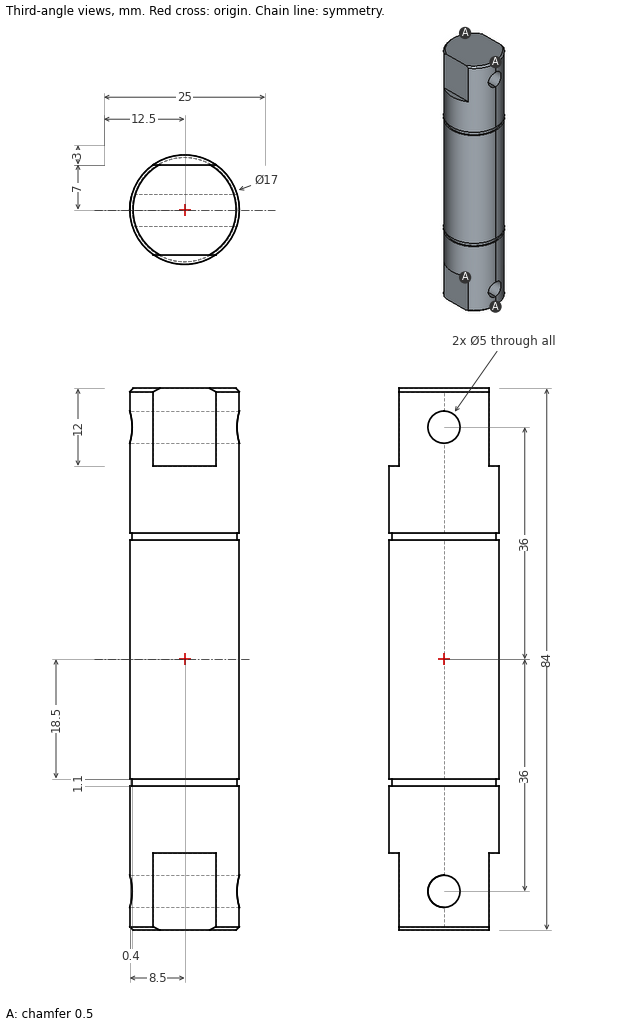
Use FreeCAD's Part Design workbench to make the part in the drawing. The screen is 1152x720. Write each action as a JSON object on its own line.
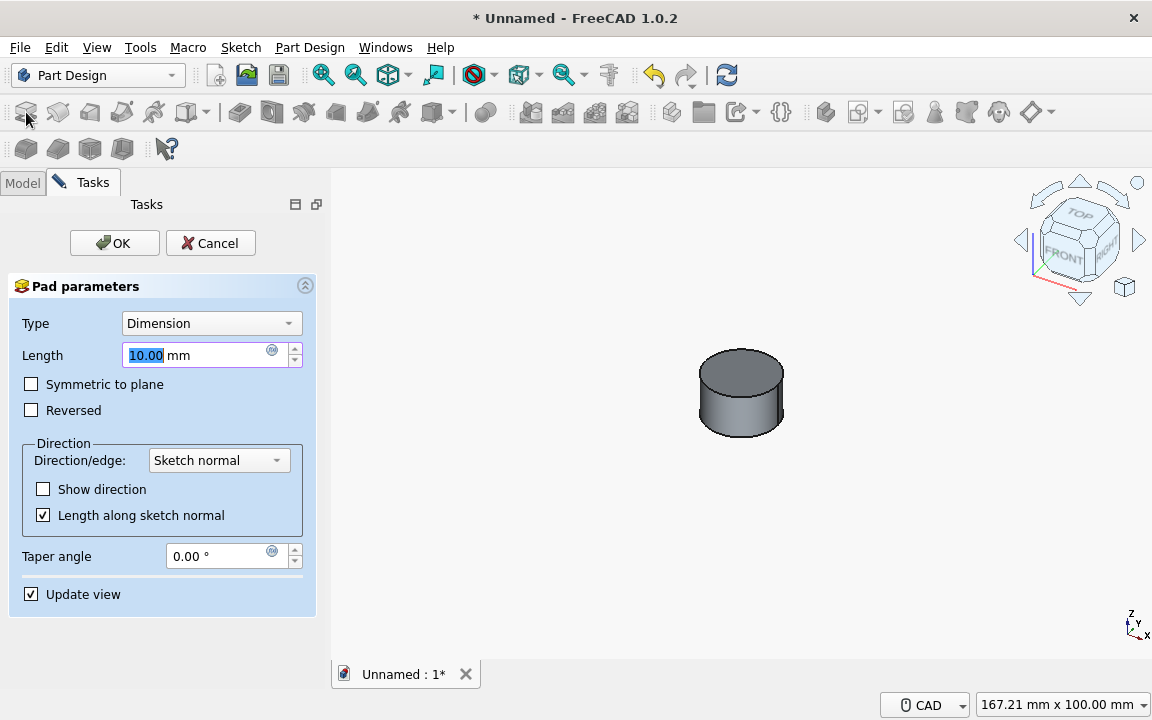
{"action": "type", "text": "84"}
{"action": "key", "text": "Tab"}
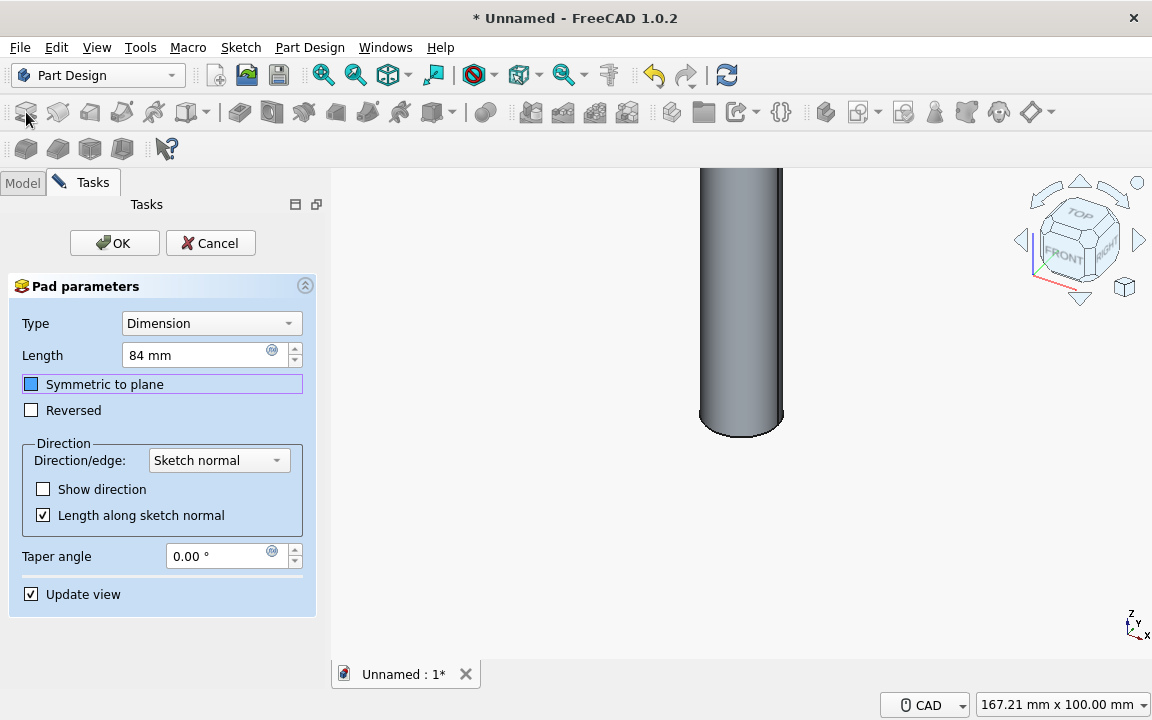
{"action": "left_click", "coordinate": [30, 384]}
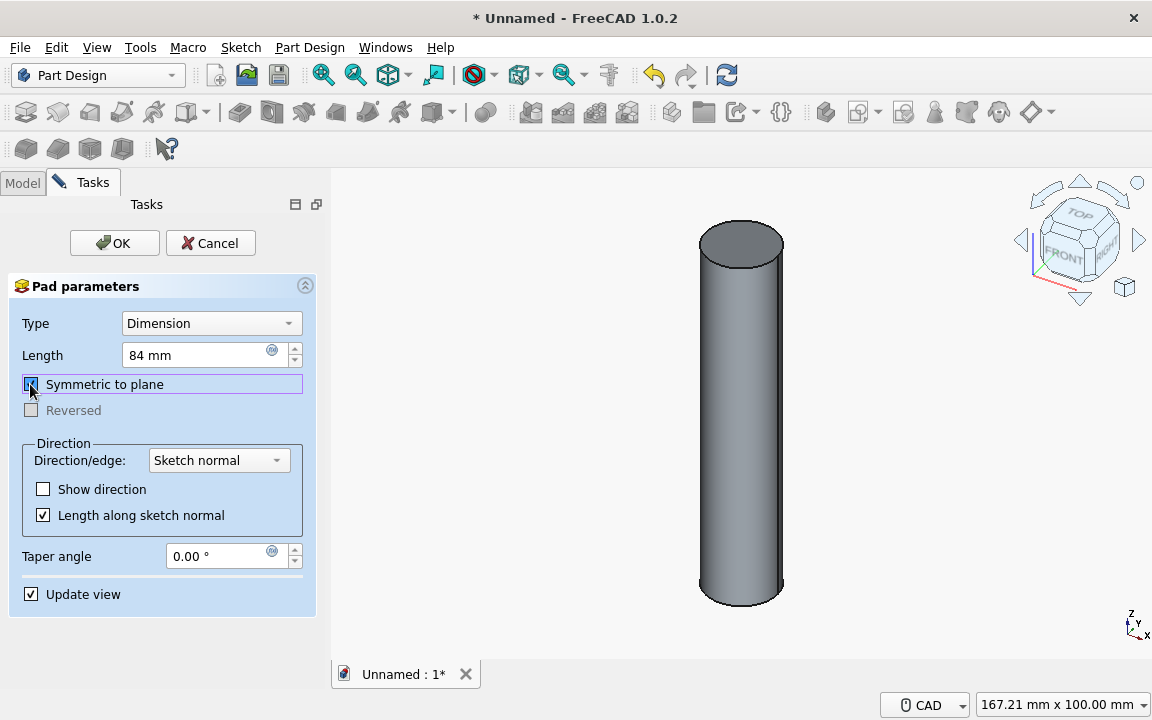
{"action": "left_click", "coordinate": [115, 243]}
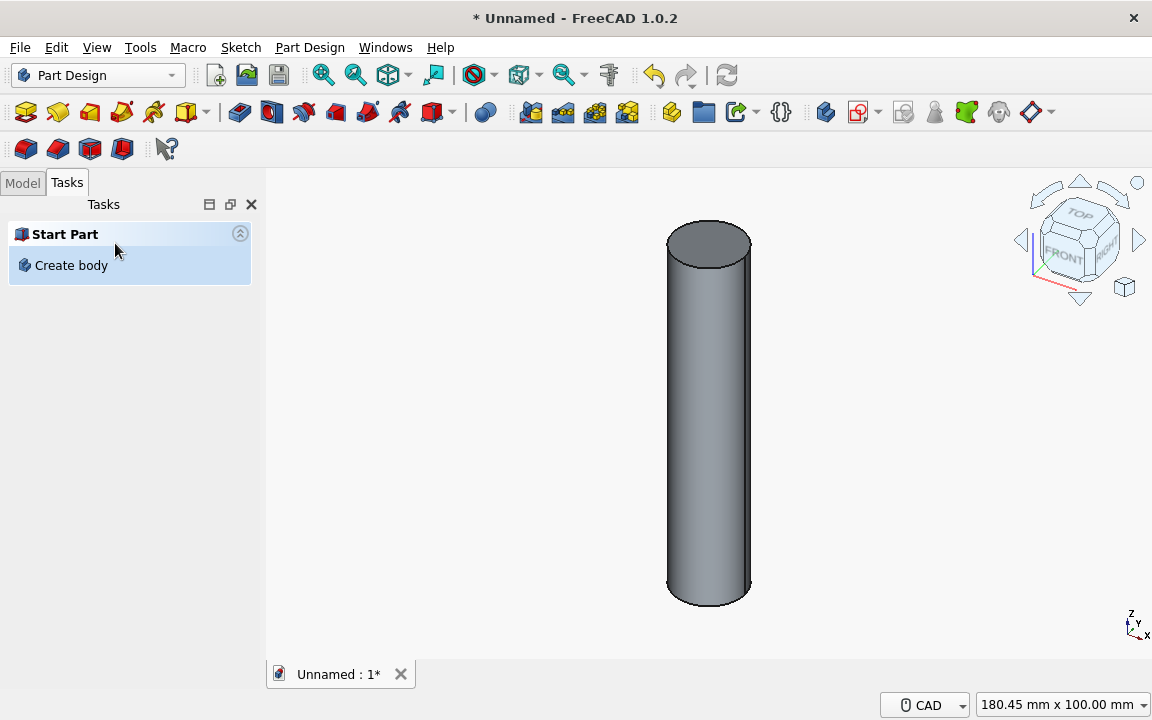
{"action": "left_click", "coordinate": [709, 244]}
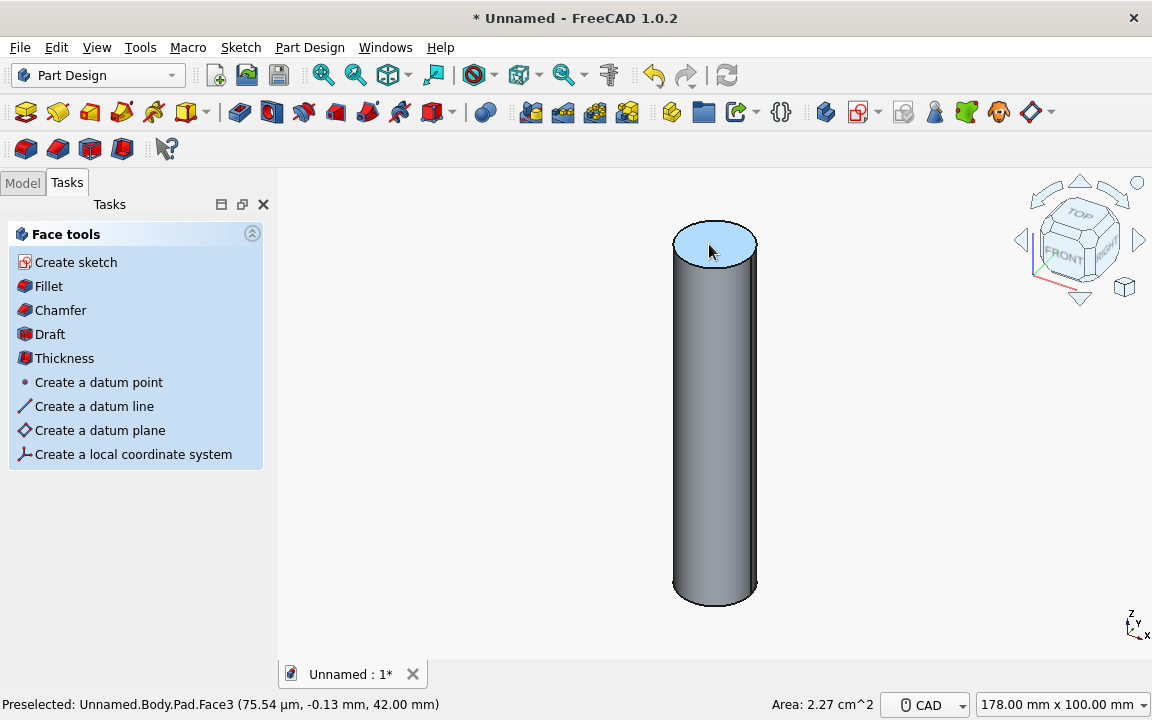
{"action": "left_click", "coordinate": [858, 112]}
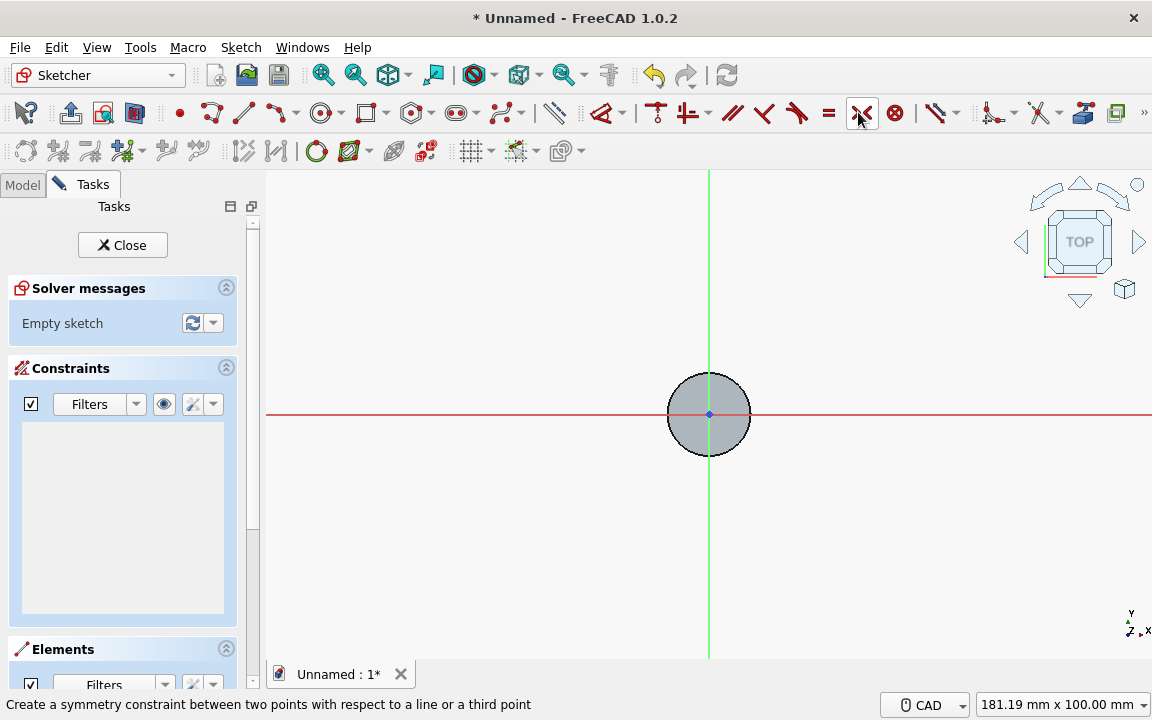
{"action": "scroll", "coordinate": [739, 415], "scroll_direction": "up", "scroll_amount": 6}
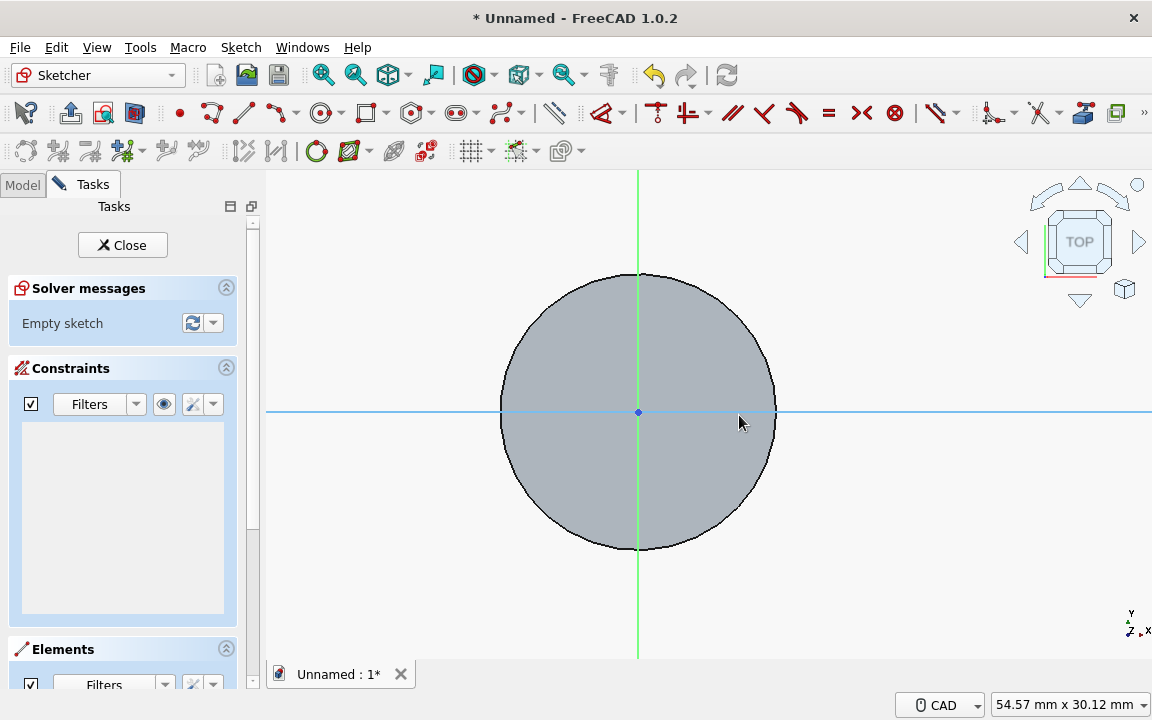
{"action": "left_click", "coordinate": [366, 114]}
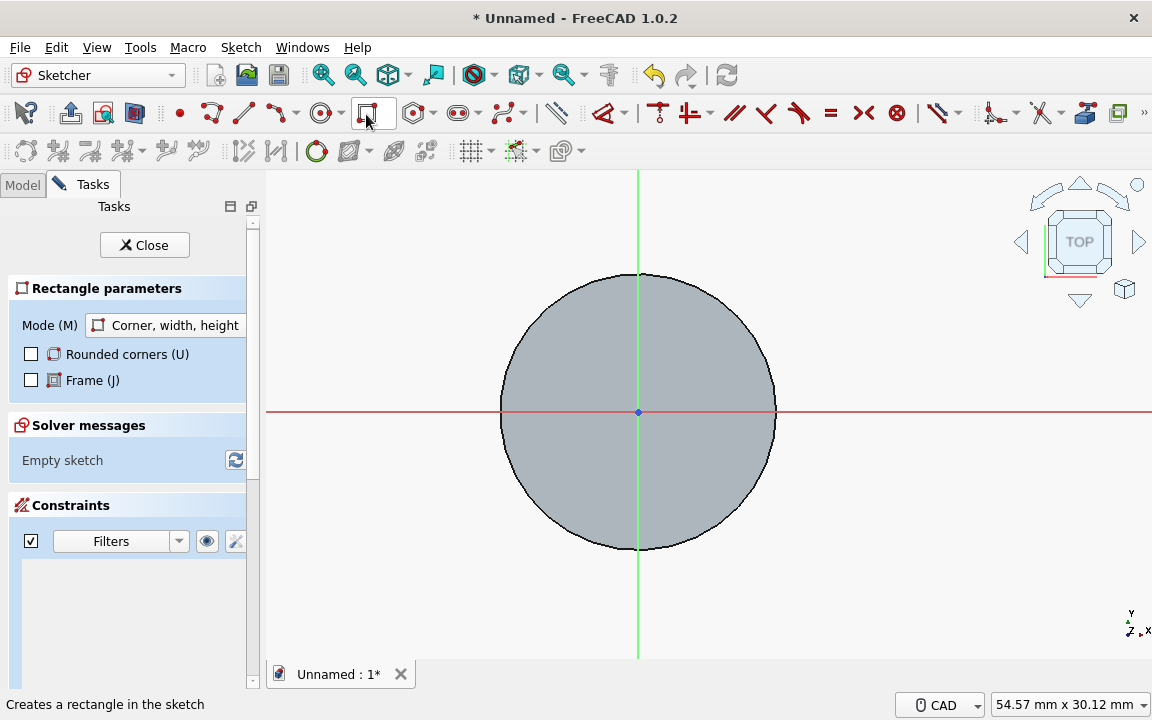
{"action": "left_click", "coordinate": [435, 250]}
{"action": "left_click", "coordinate": [841, 299]}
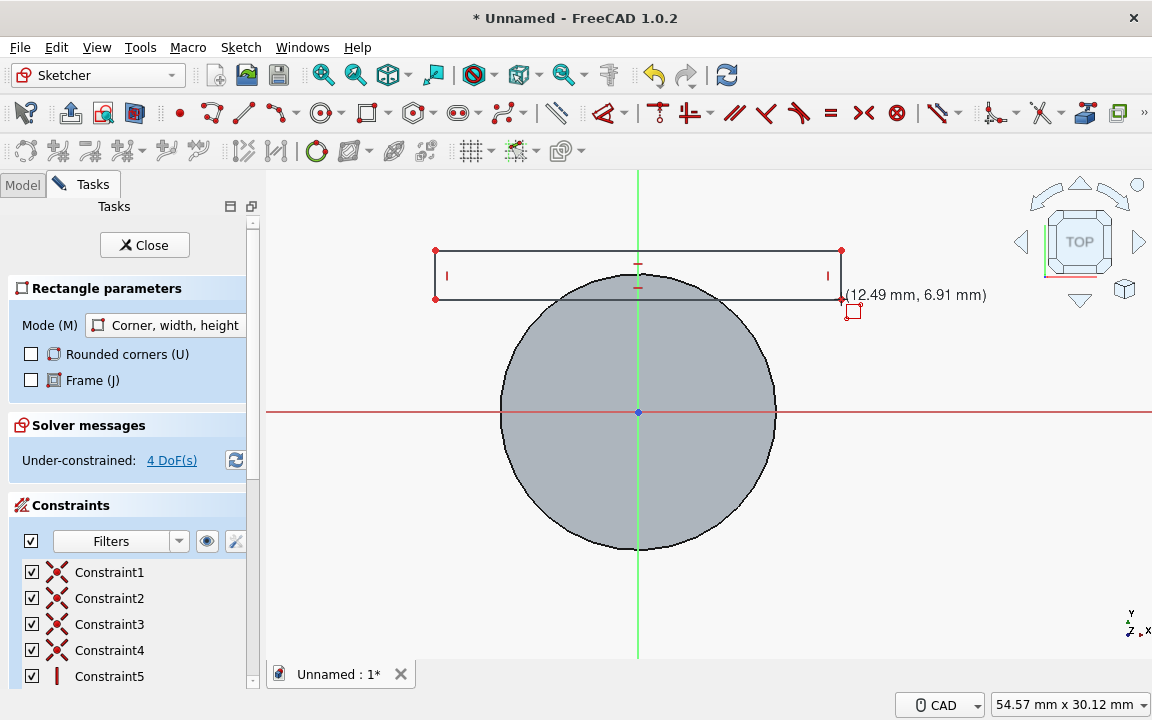
{"action": "left_click", "coordinate": [435, 526]}
{"action": "left_click", "coordinate": [841, 575]}
{"action": "key", "text": "Escape"}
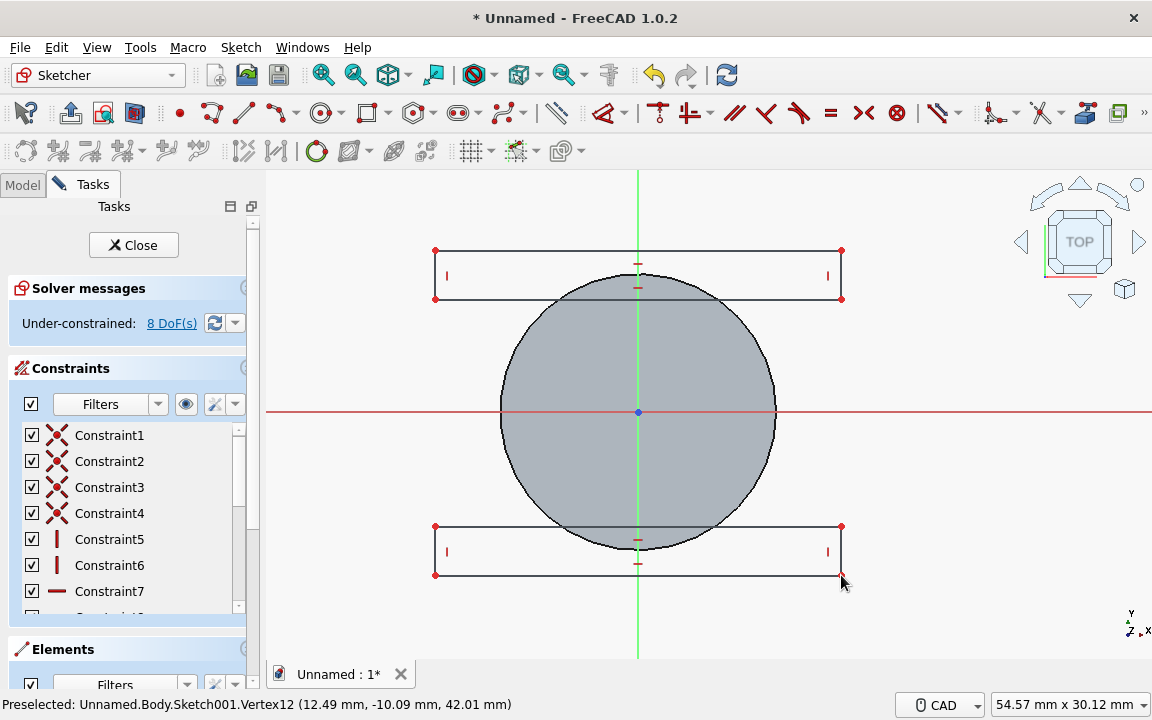
{"action": "left_click", "coordinate": [435, 300]}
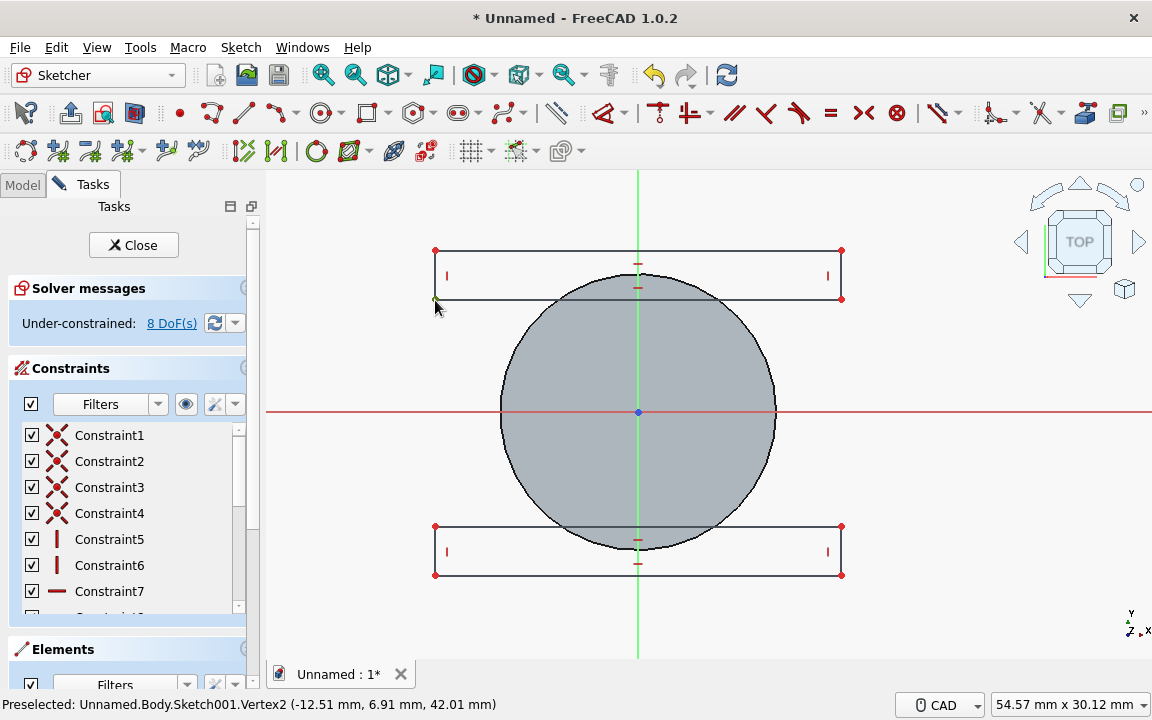
{"action": "left_click", "coordinate": [435, 527]}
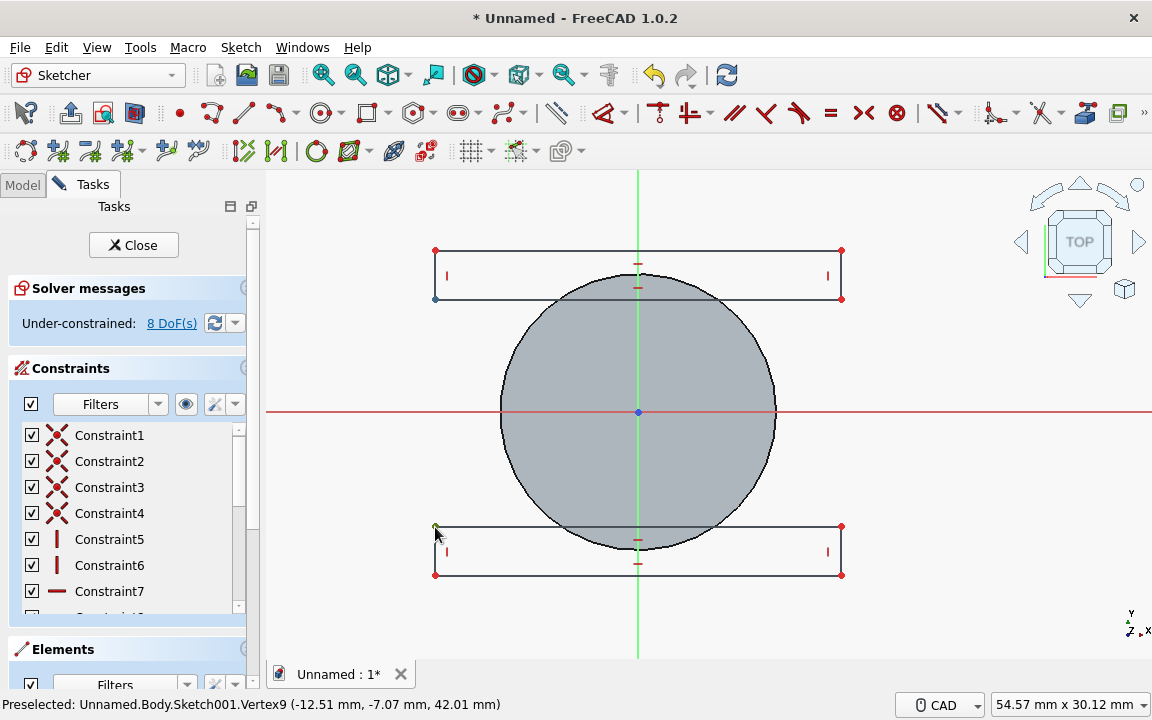
{"action": "left_click", "coordinate": [344, 412]}